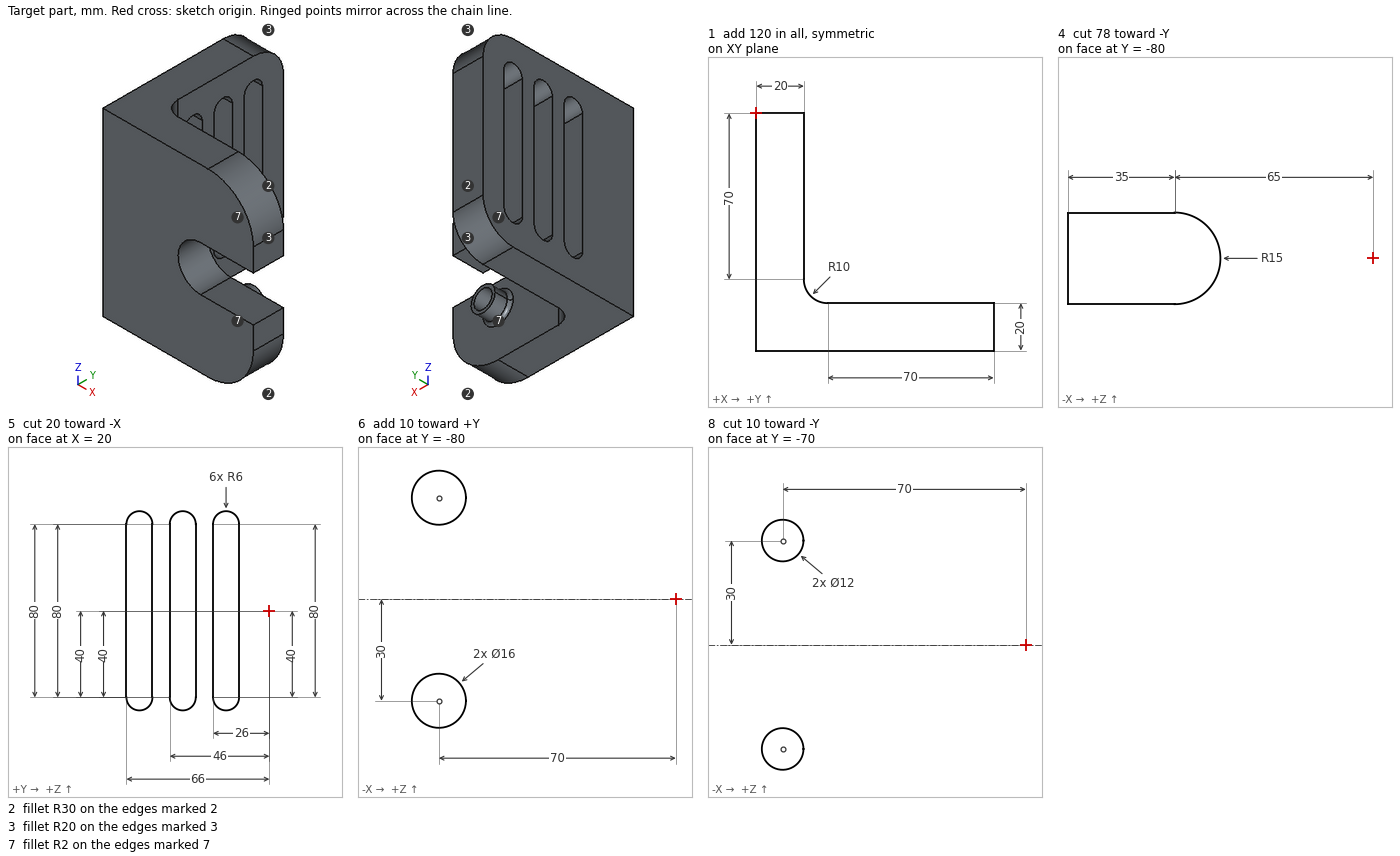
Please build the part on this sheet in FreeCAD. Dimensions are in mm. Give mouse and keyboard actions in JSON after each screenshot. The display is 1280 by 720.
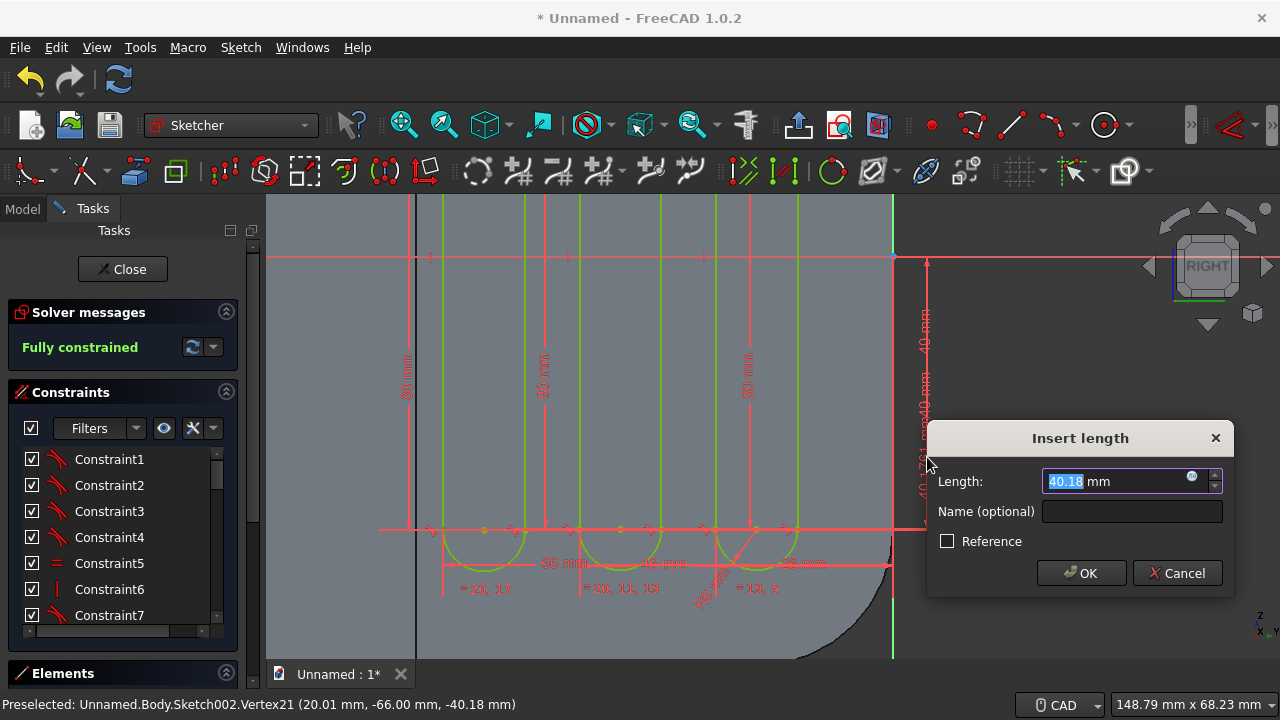
{"action": "type", "text": "40"}
{"action": "key", "text": "Return"}
{"action": "key", "text": "Escape"}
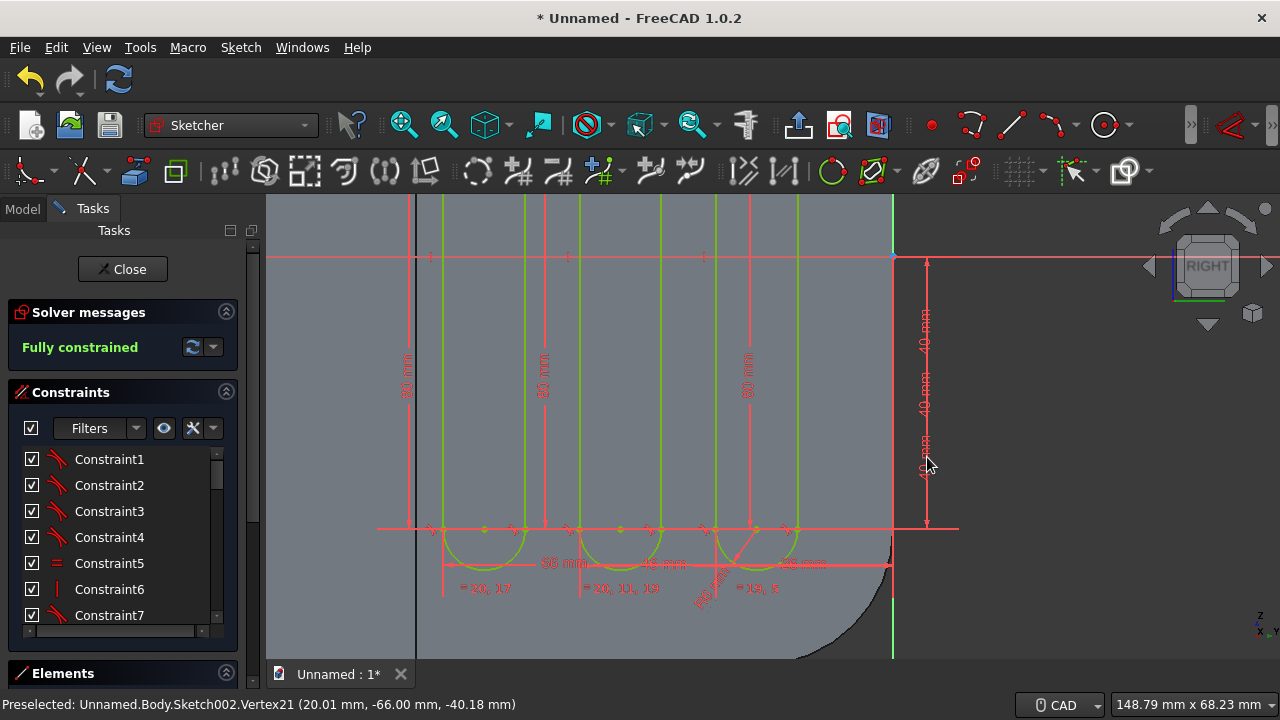
{"action": "left_click", "coordinate": [123, 269]}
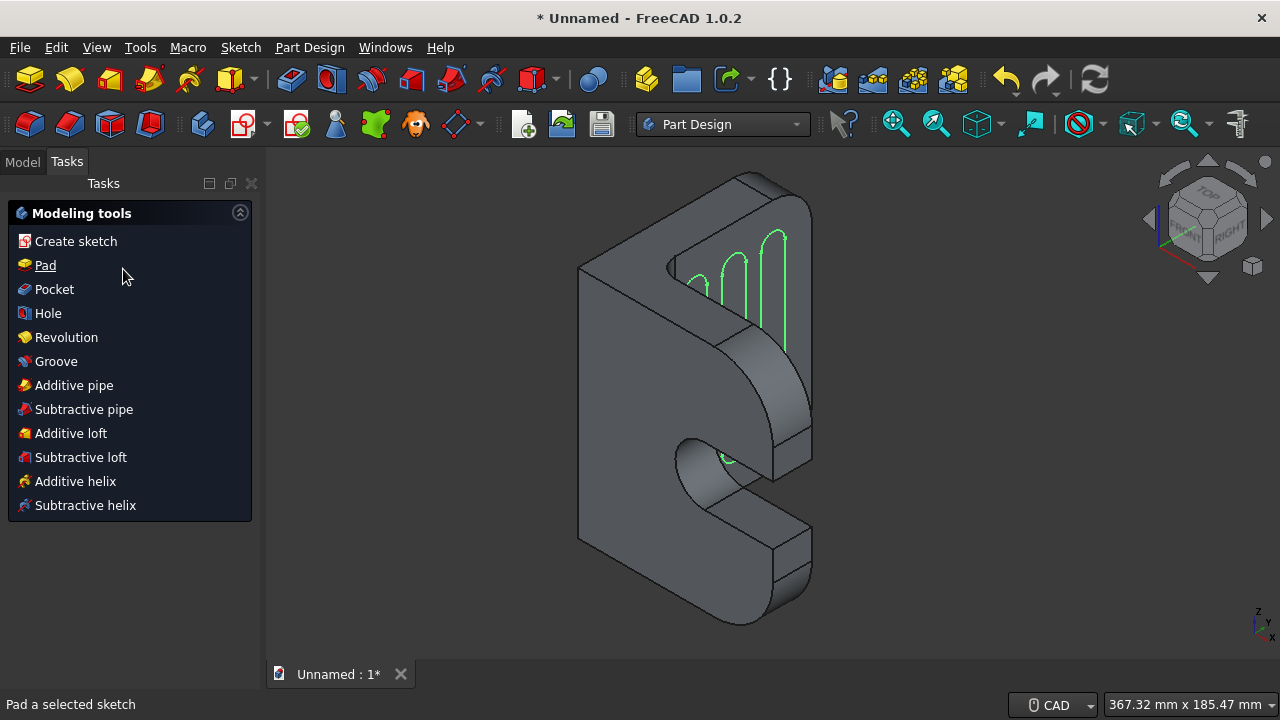
{"action": "left_click", "coordinate": [292, 80]}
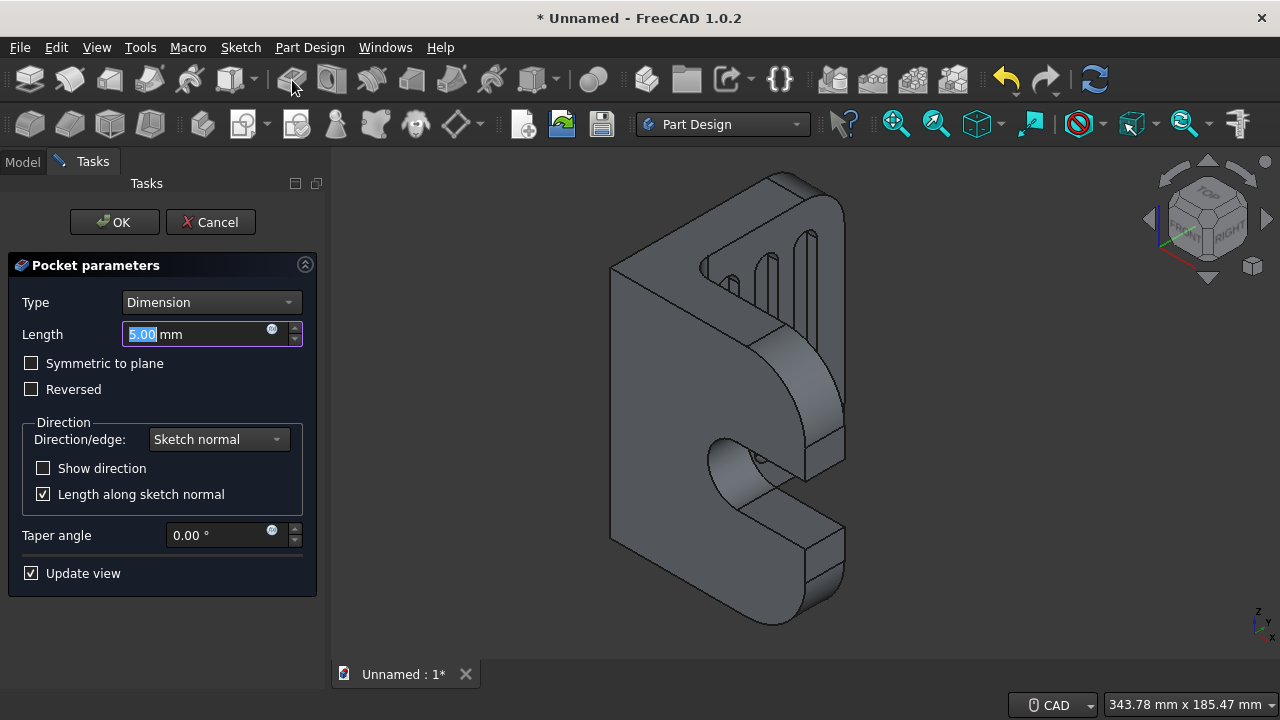
{"action": "type", "text": "20"}
{"action": "key", "text": "Tab"}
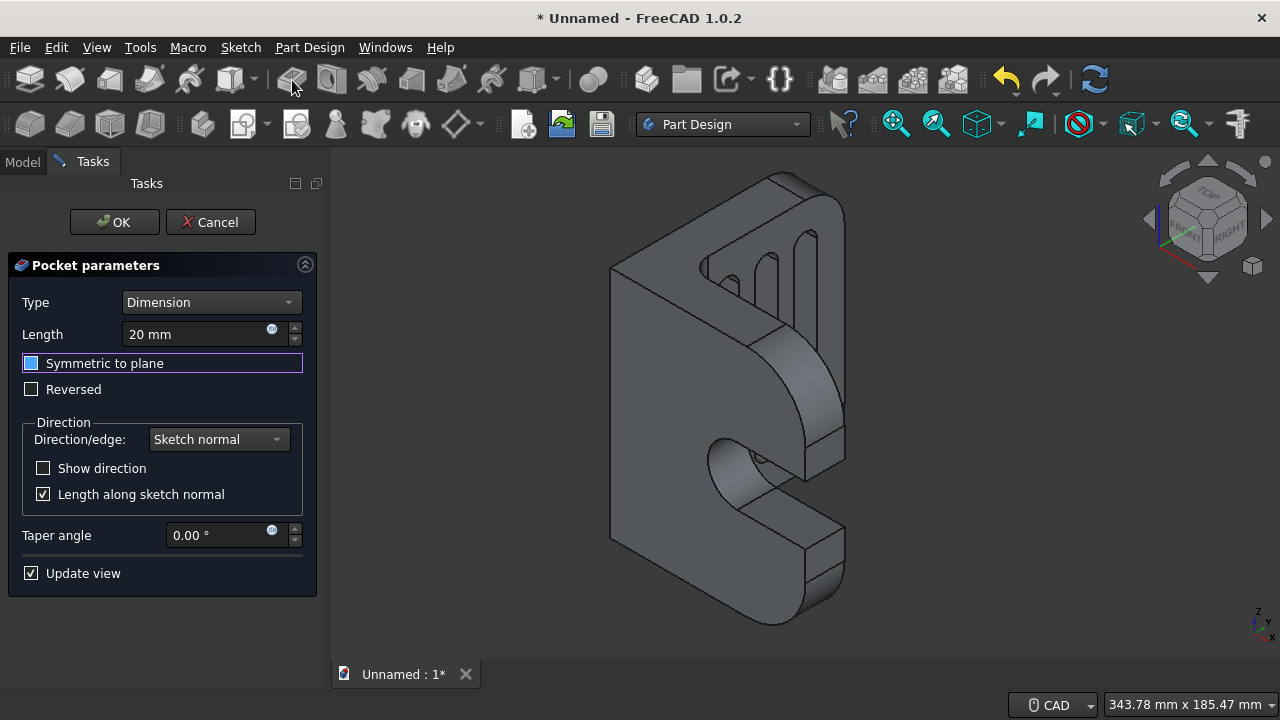
{"action": "left_click", "coordinate": [115, 222]}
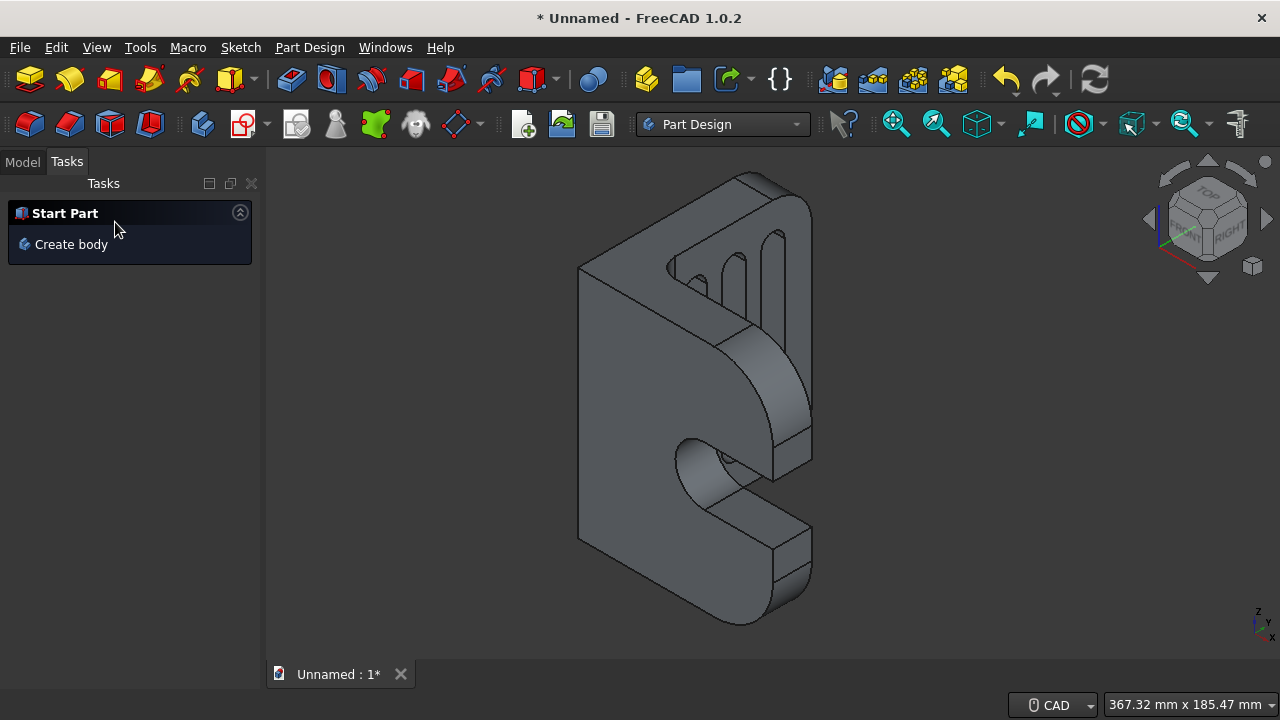
{"action": "key", "text": "4"}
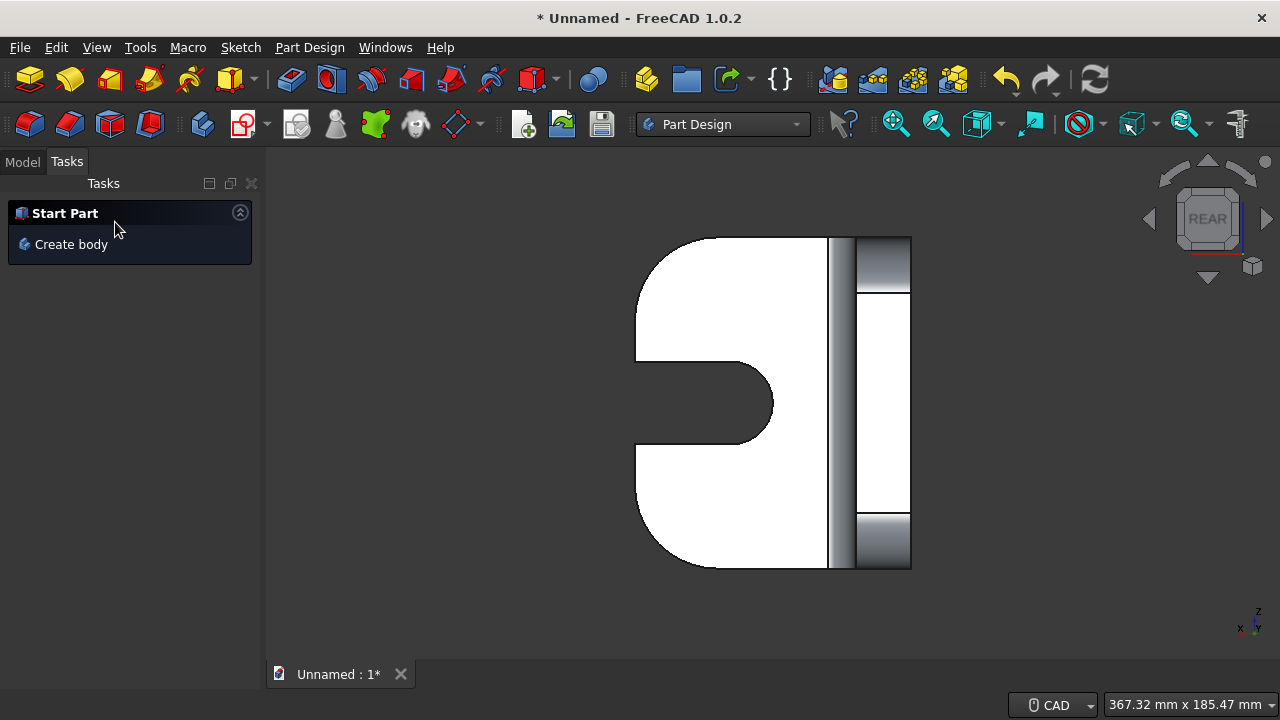
{"action": "left_click", "coordinate": [759, 497]}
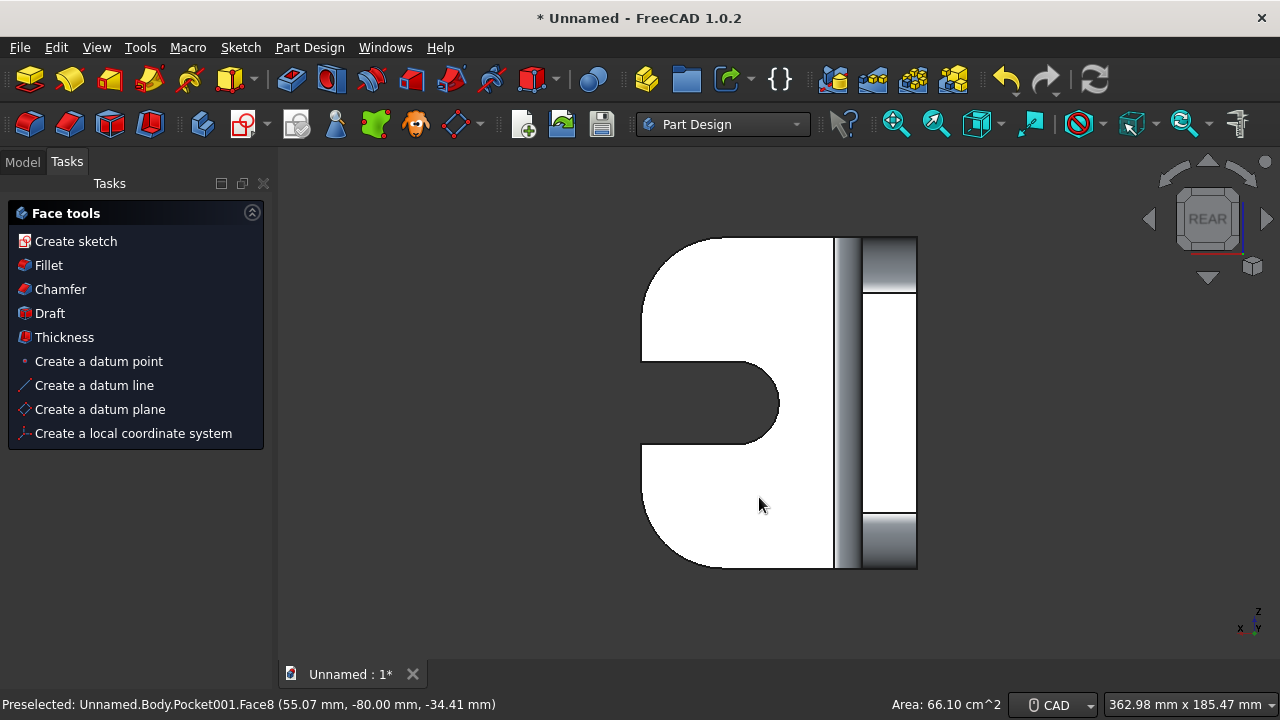
{"action": "left_click", "coordinate": [244, 124]}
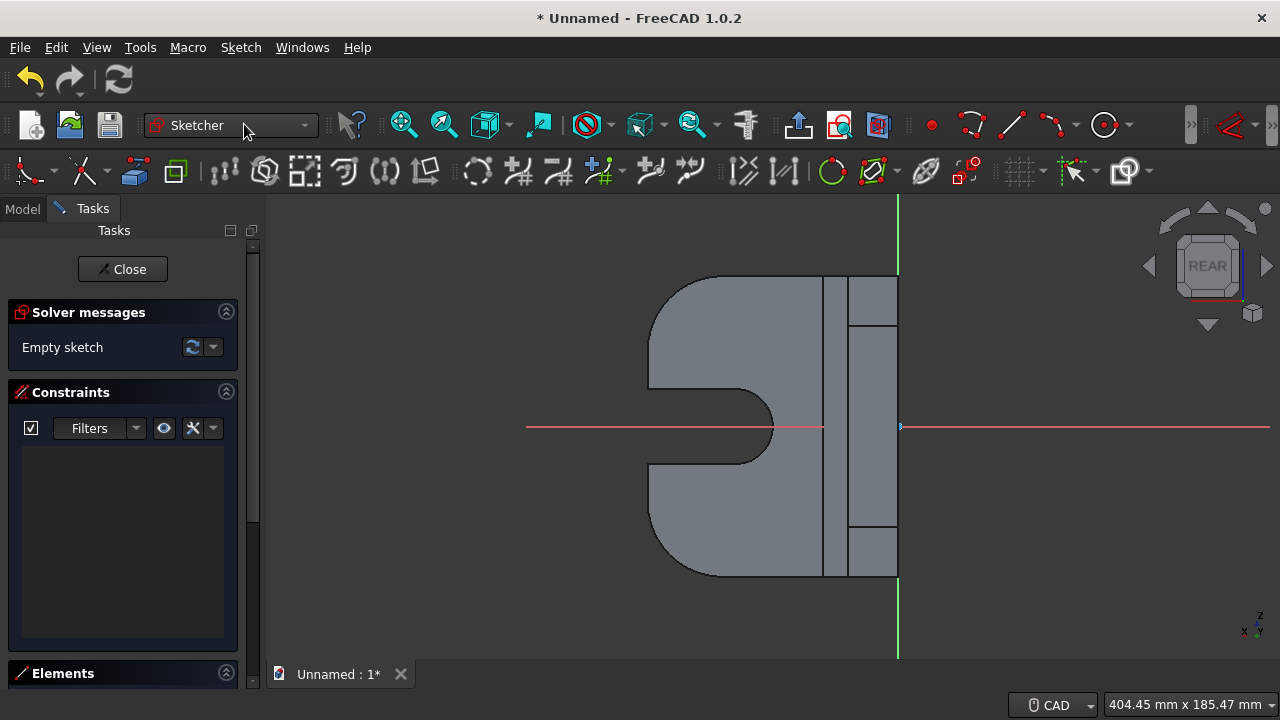
{"action": "key", "text": "q s"}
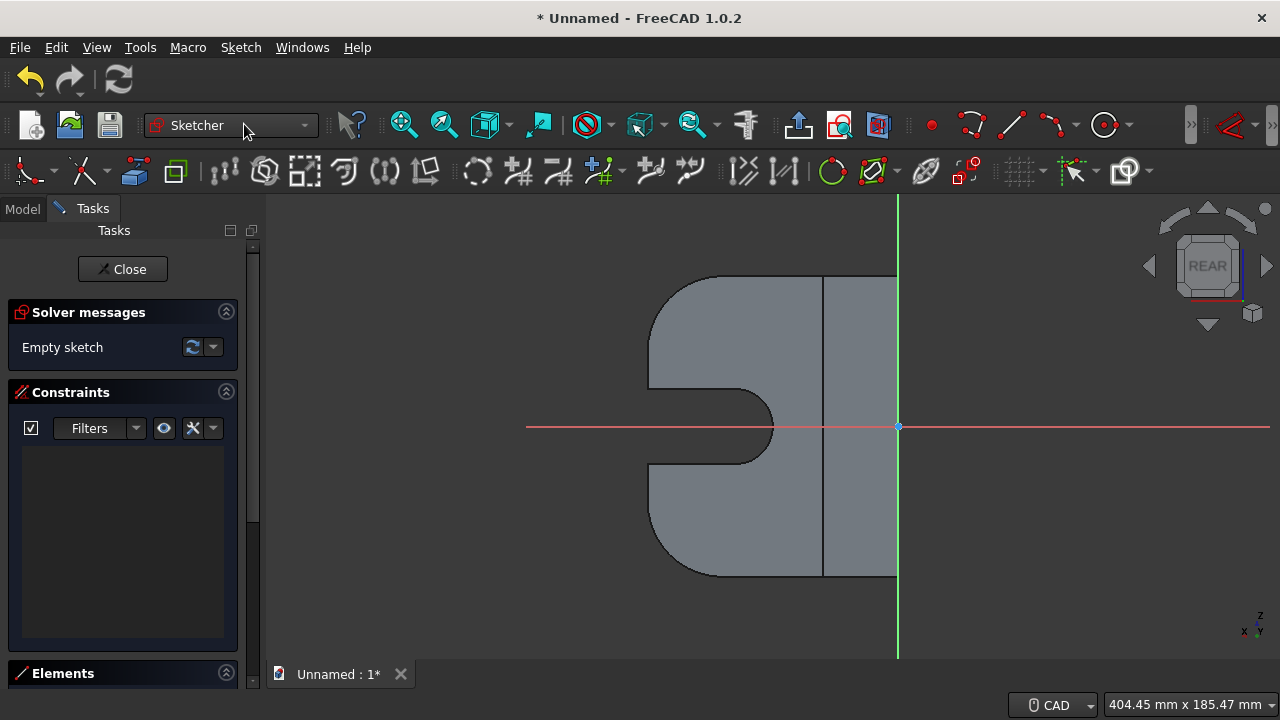
{"action": "scroll", "coordinate": [996, 426], "scroll_direction": "up", "scroll_amount": 2}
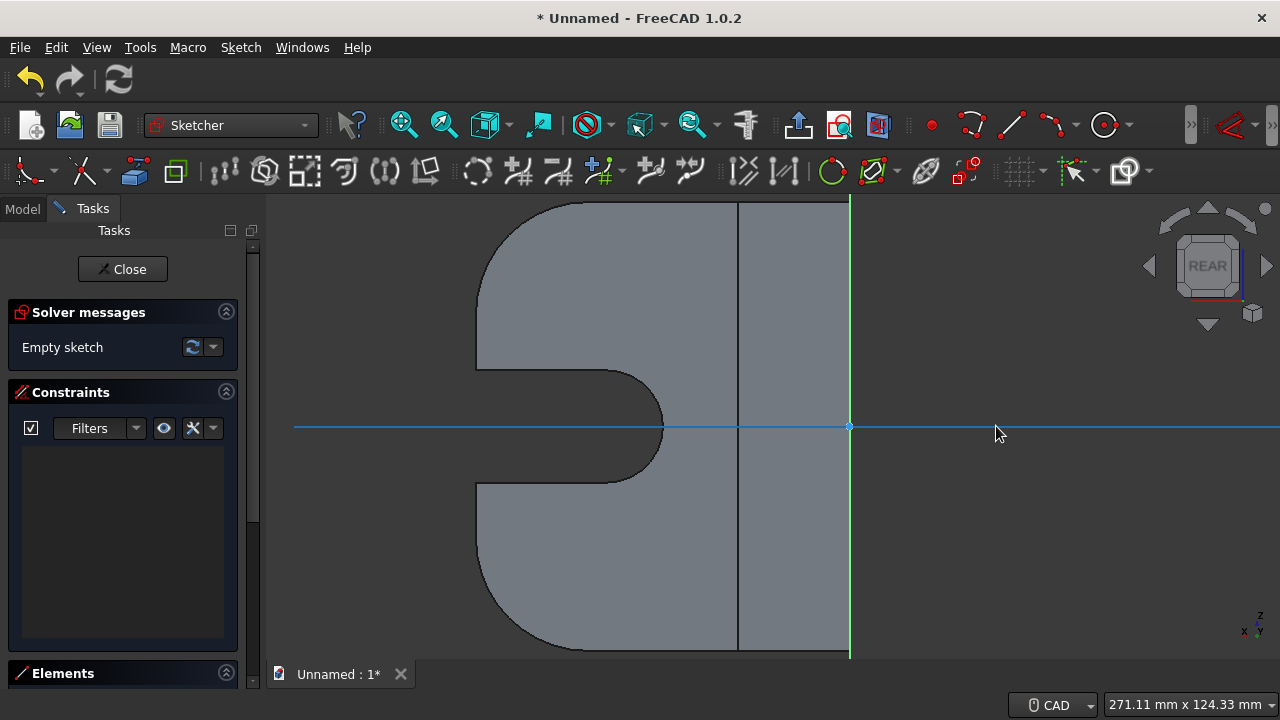
{"action": "key", "text": "g c"}